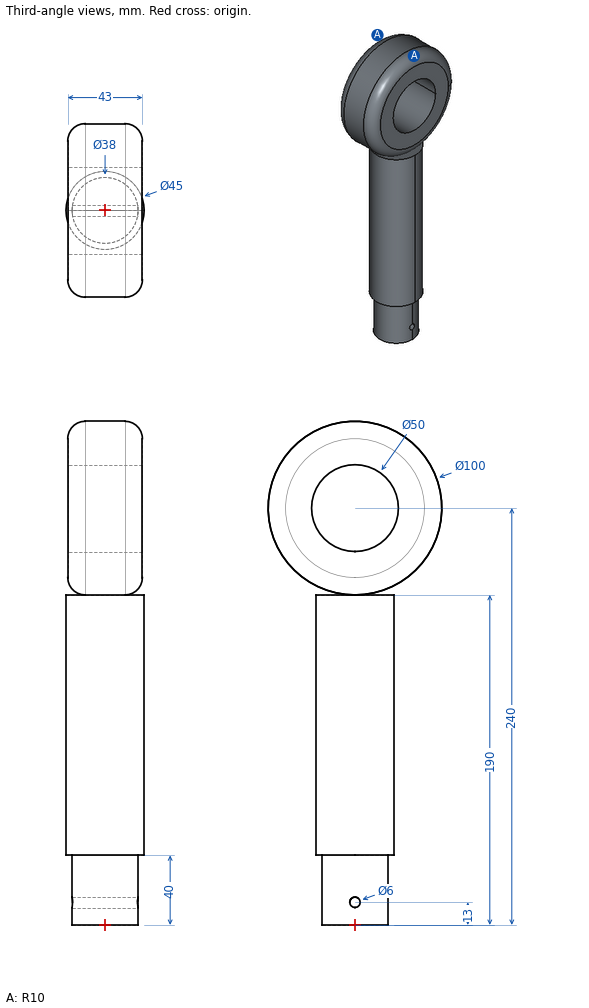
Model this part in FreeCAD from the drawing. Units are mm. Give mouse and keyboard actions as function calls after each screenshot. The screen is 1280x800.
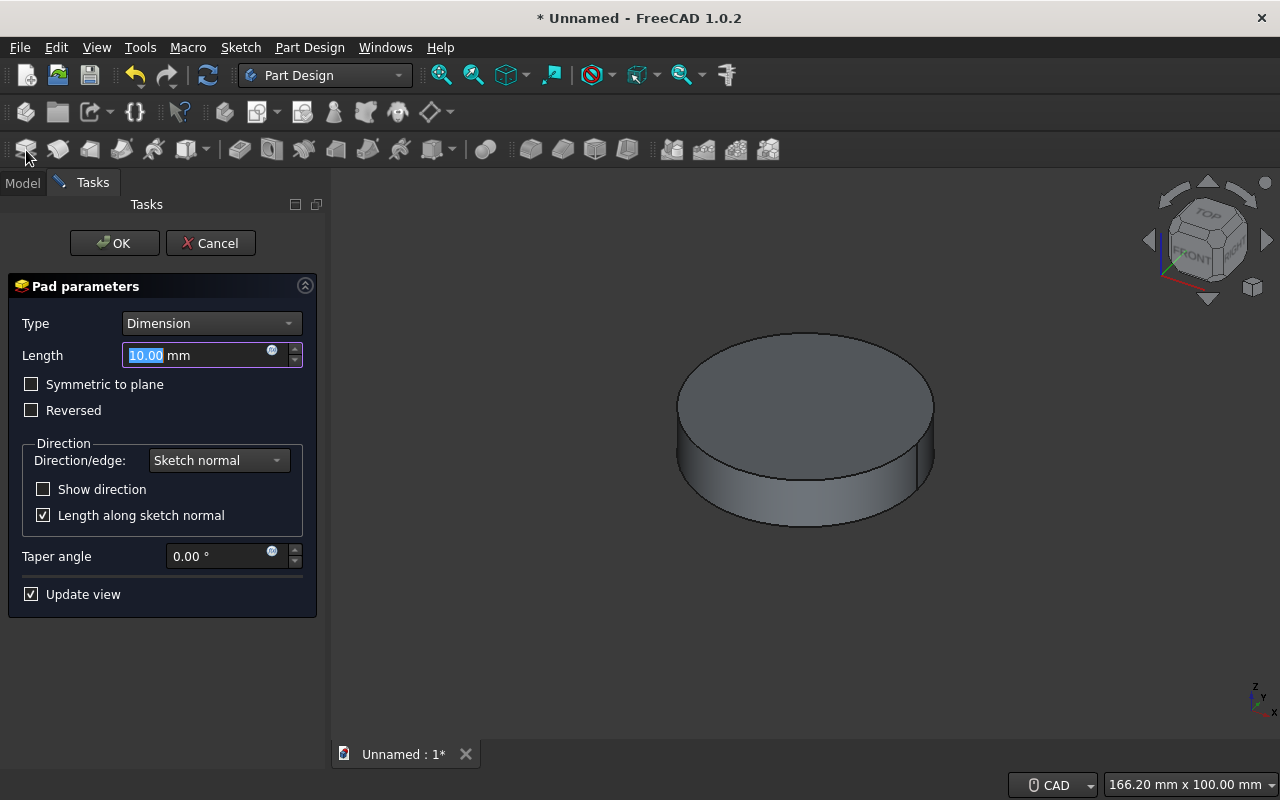
text(190)
key(Tab)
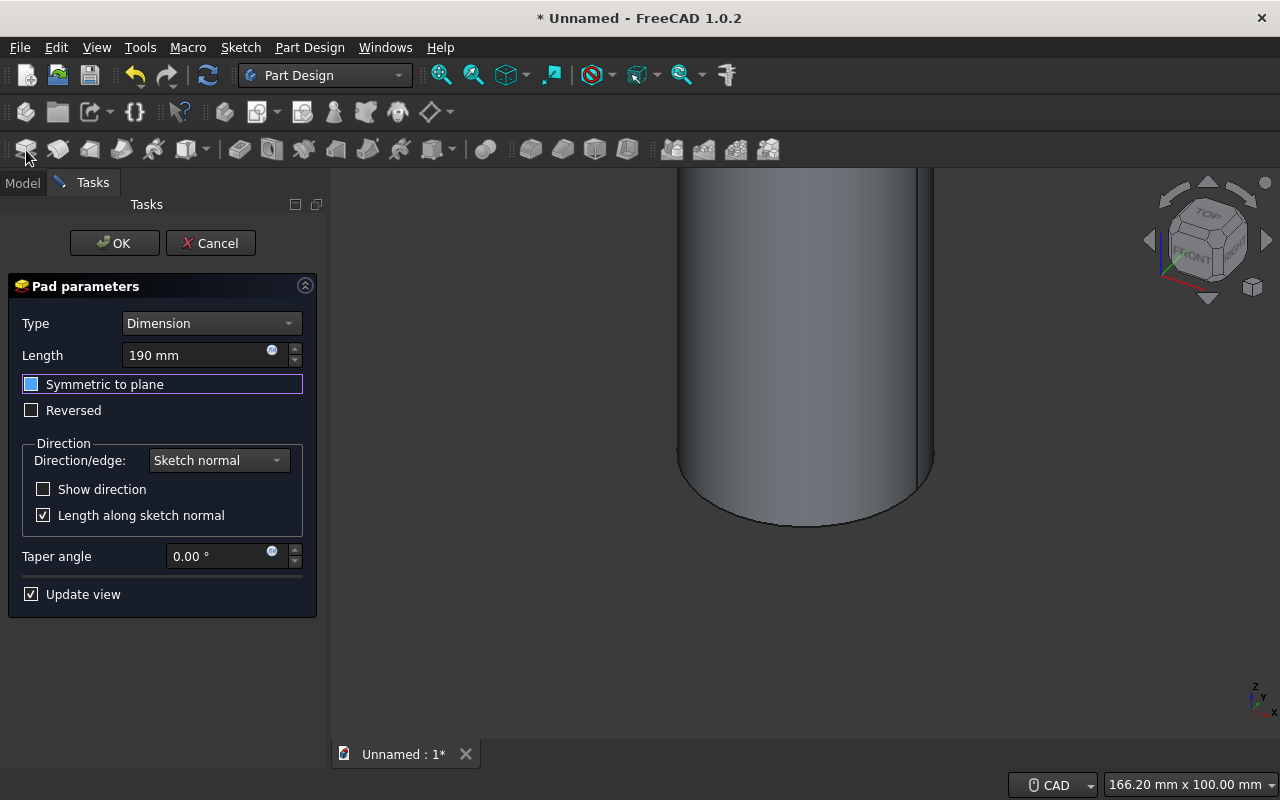
click(115, 243)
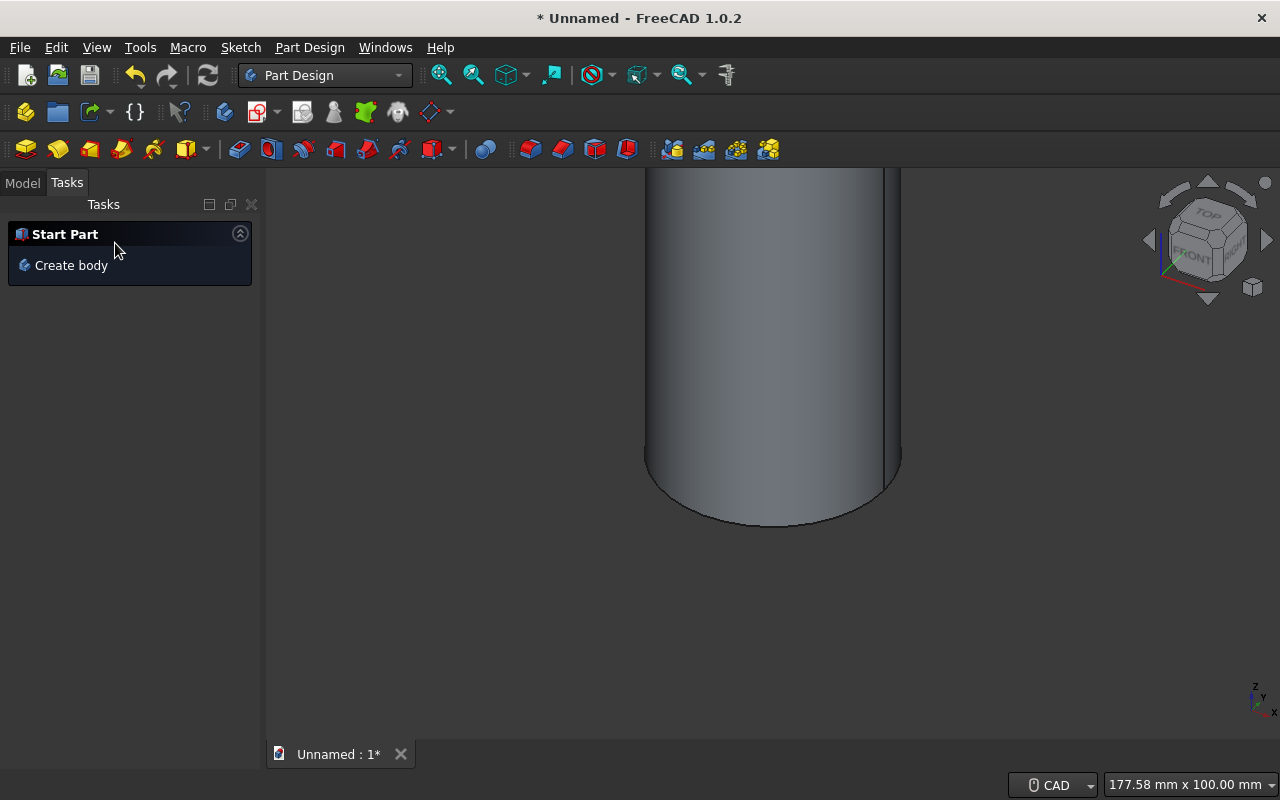
key(v)
key(f)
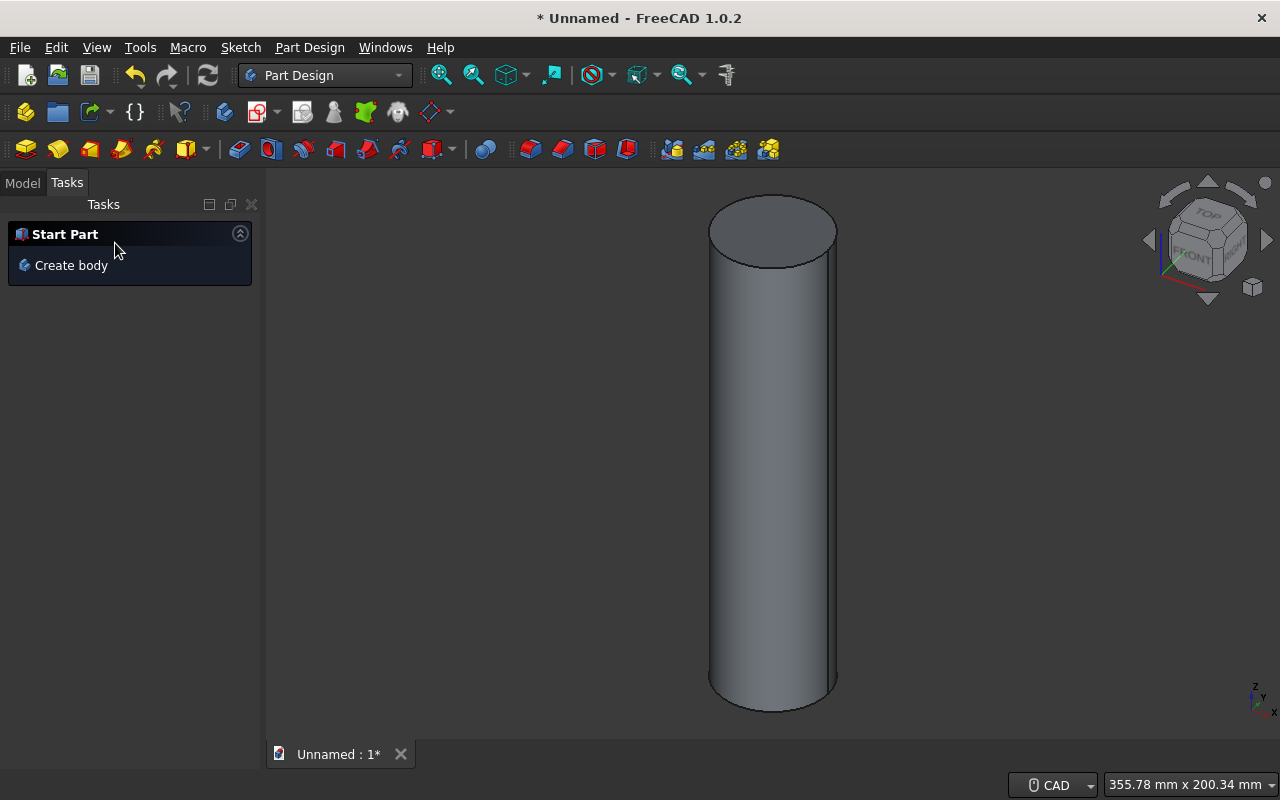
click(258, 112)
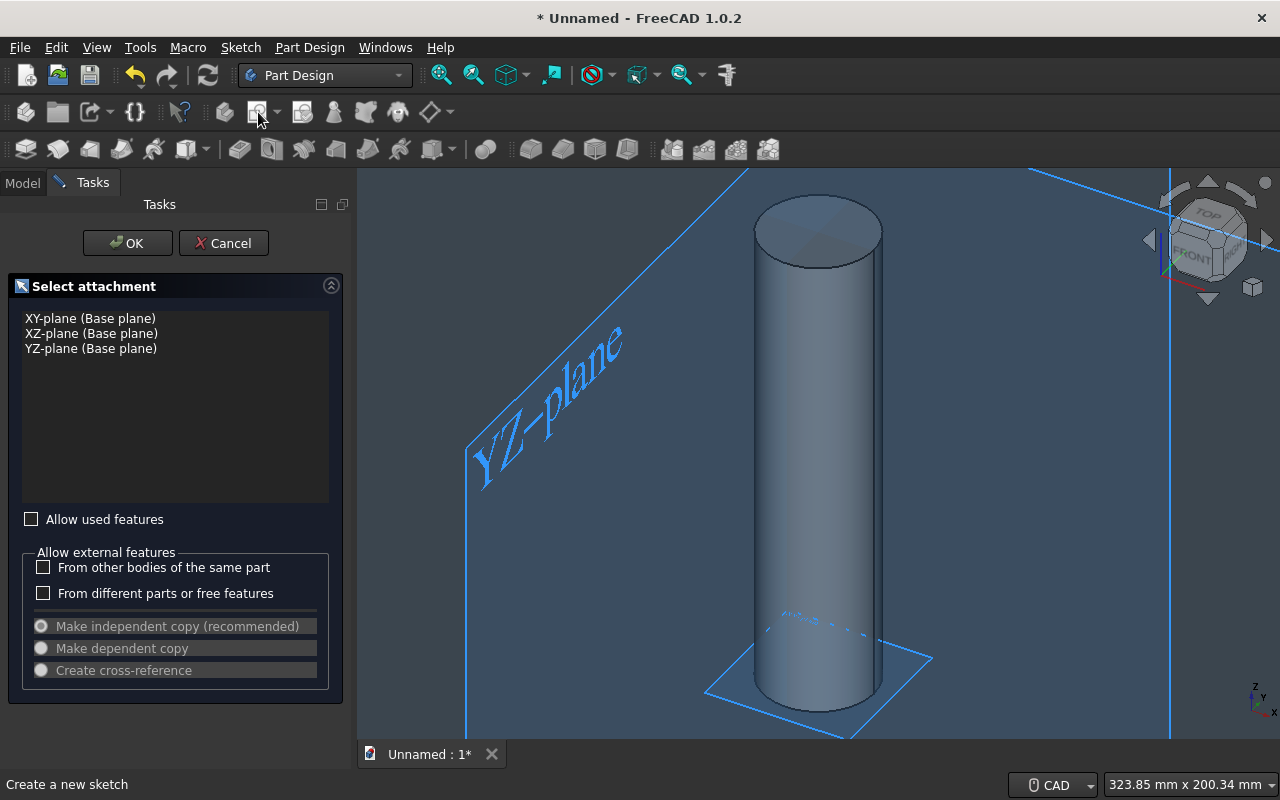
click(82, 318)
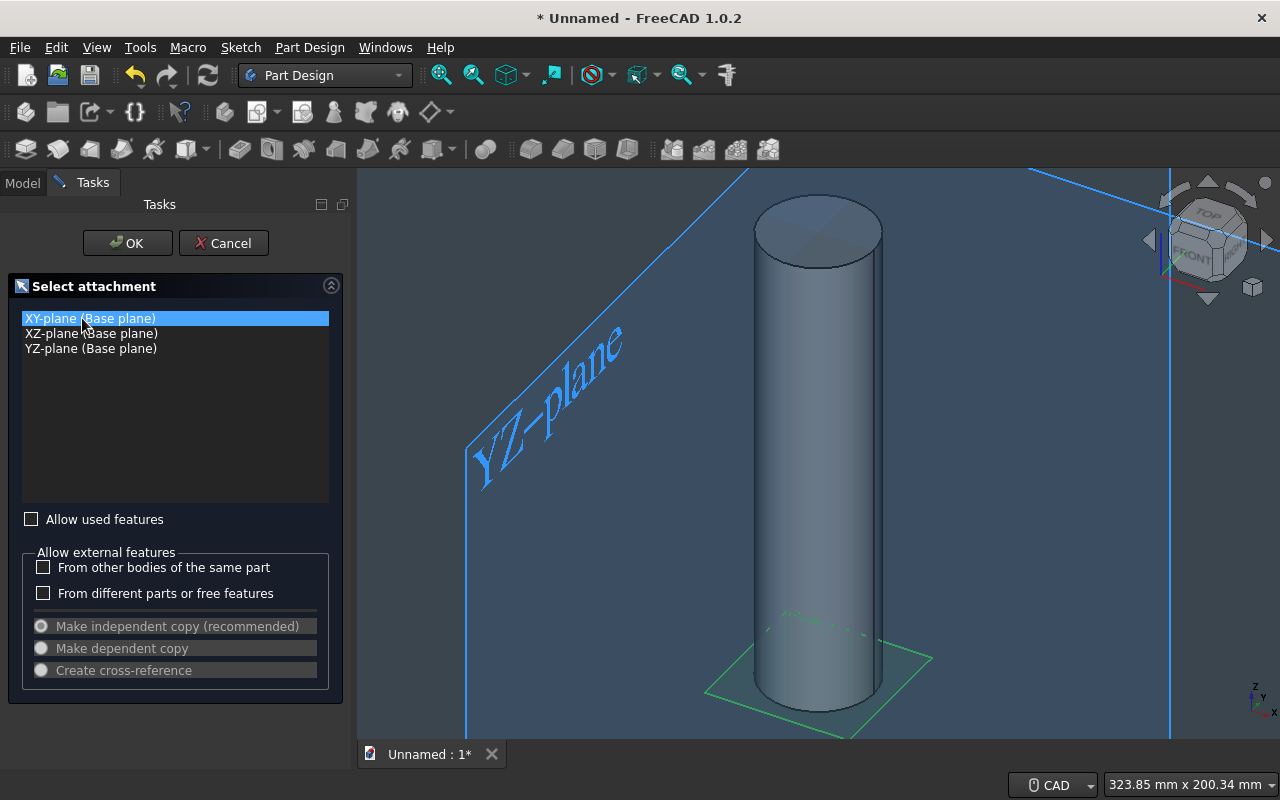
click(128, 243)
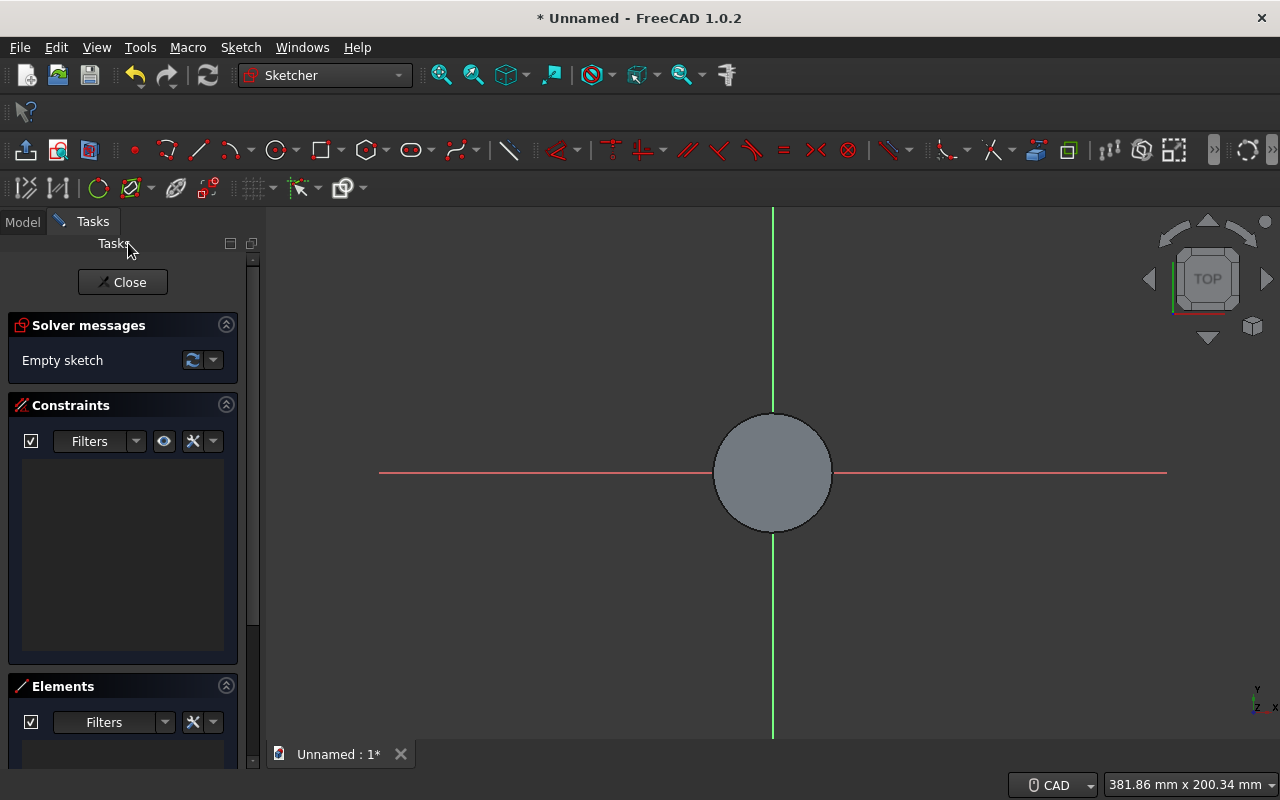
click(90, 150)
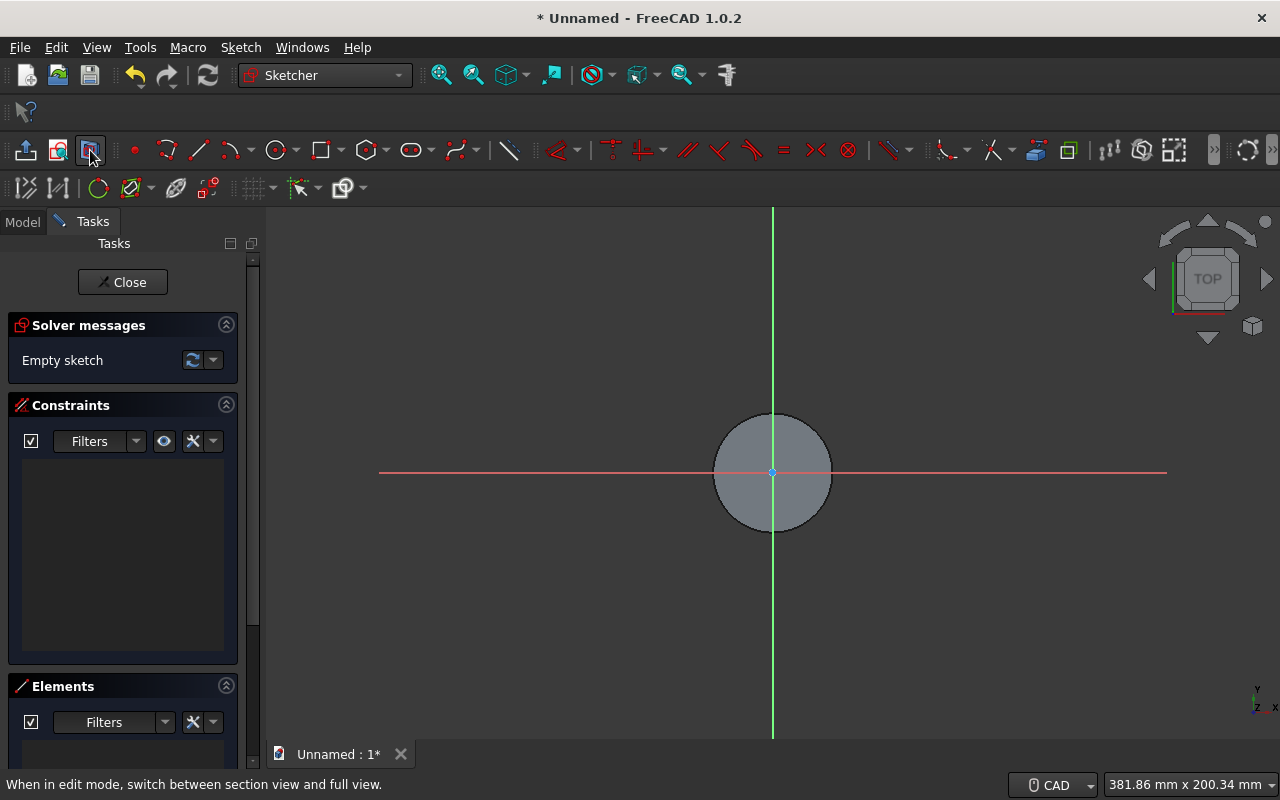
scroll(813, 473, up, 5)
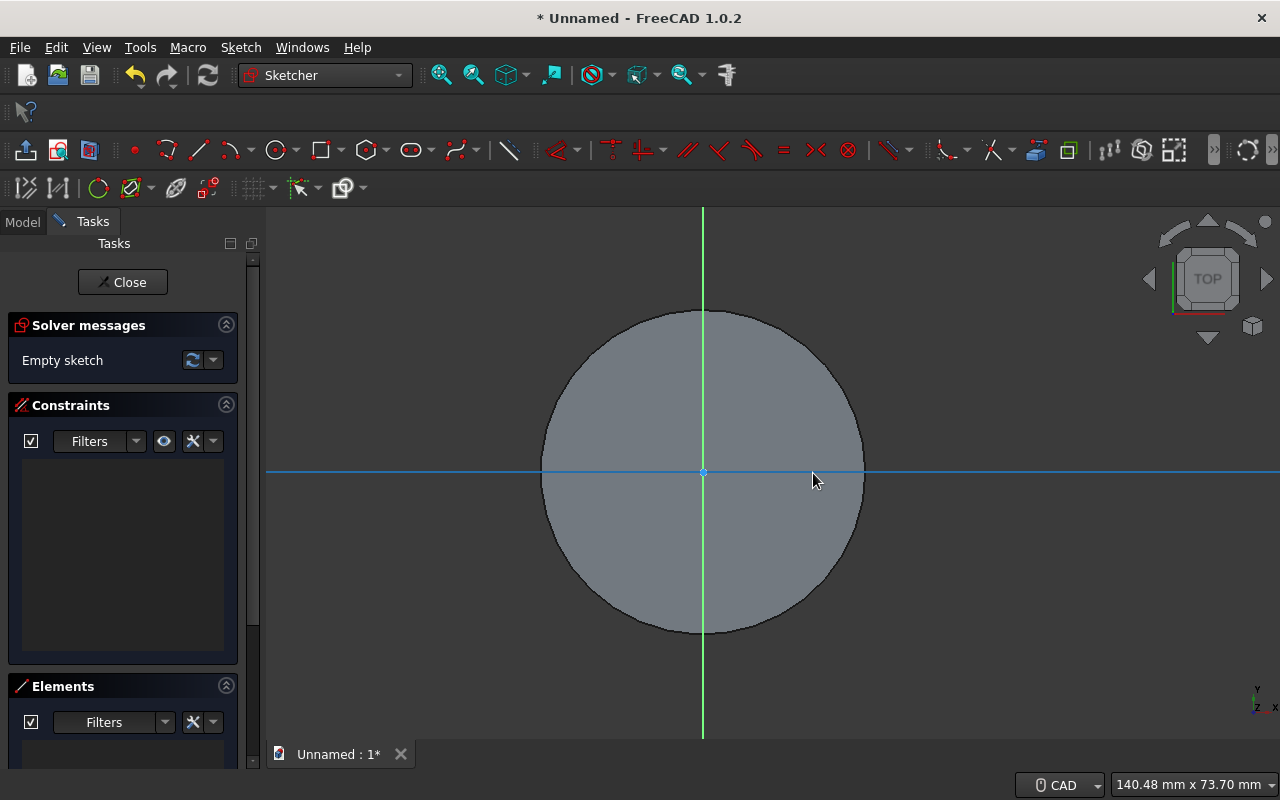
key(g)
key(c)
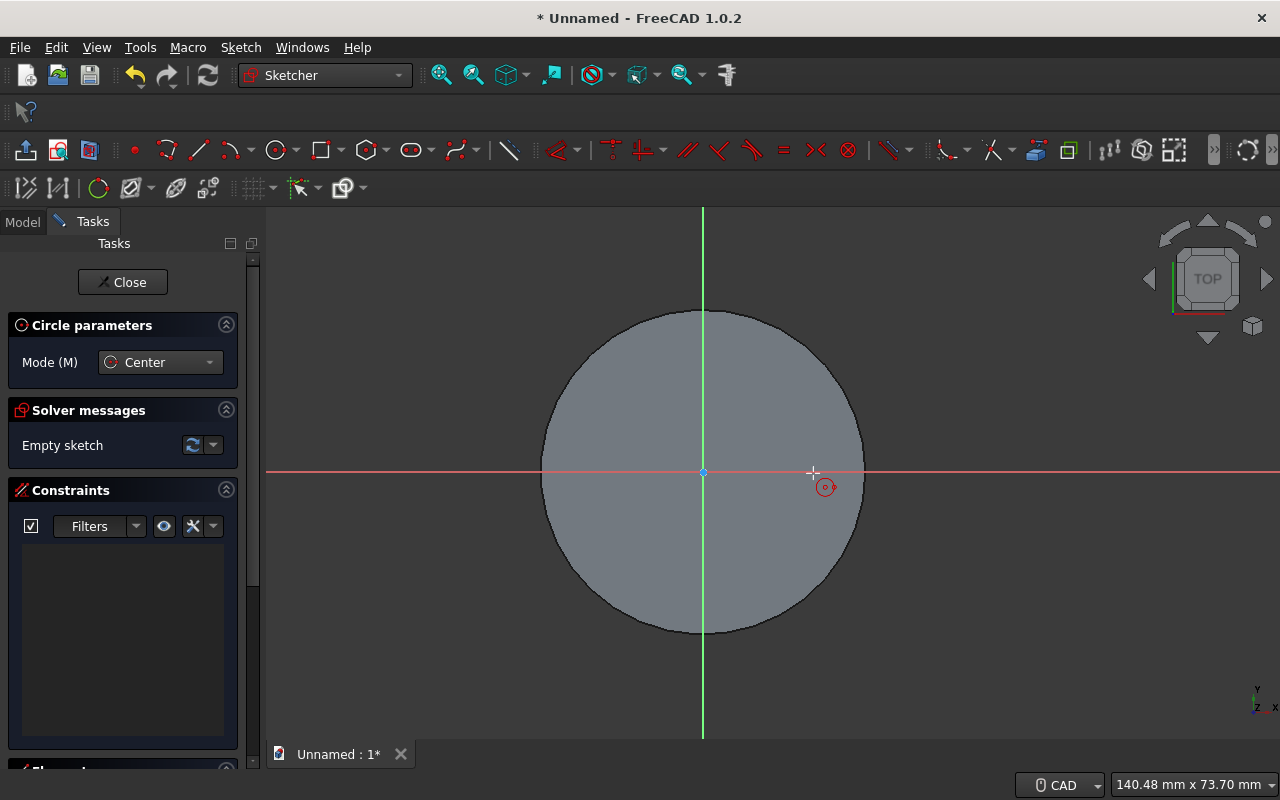
click(703, 472)
move(818, 357)